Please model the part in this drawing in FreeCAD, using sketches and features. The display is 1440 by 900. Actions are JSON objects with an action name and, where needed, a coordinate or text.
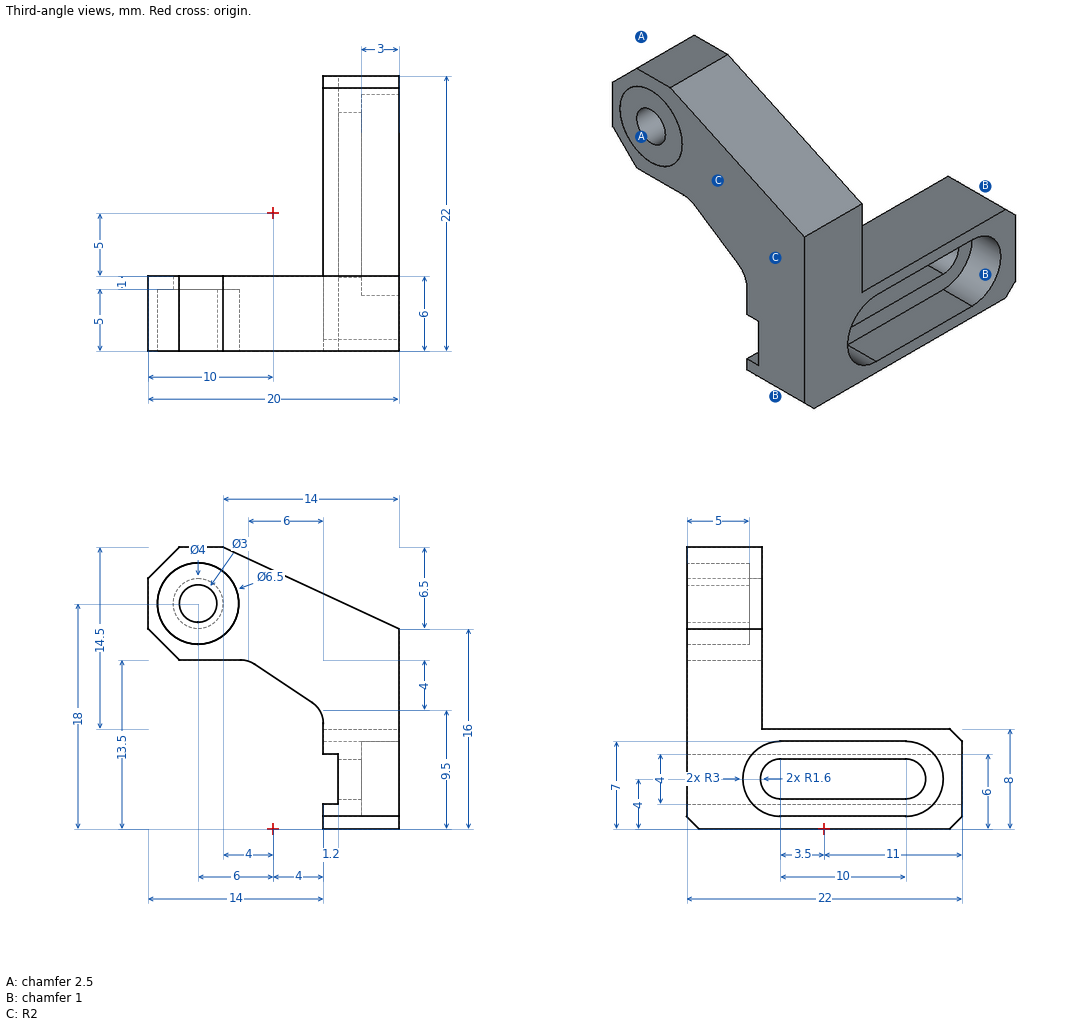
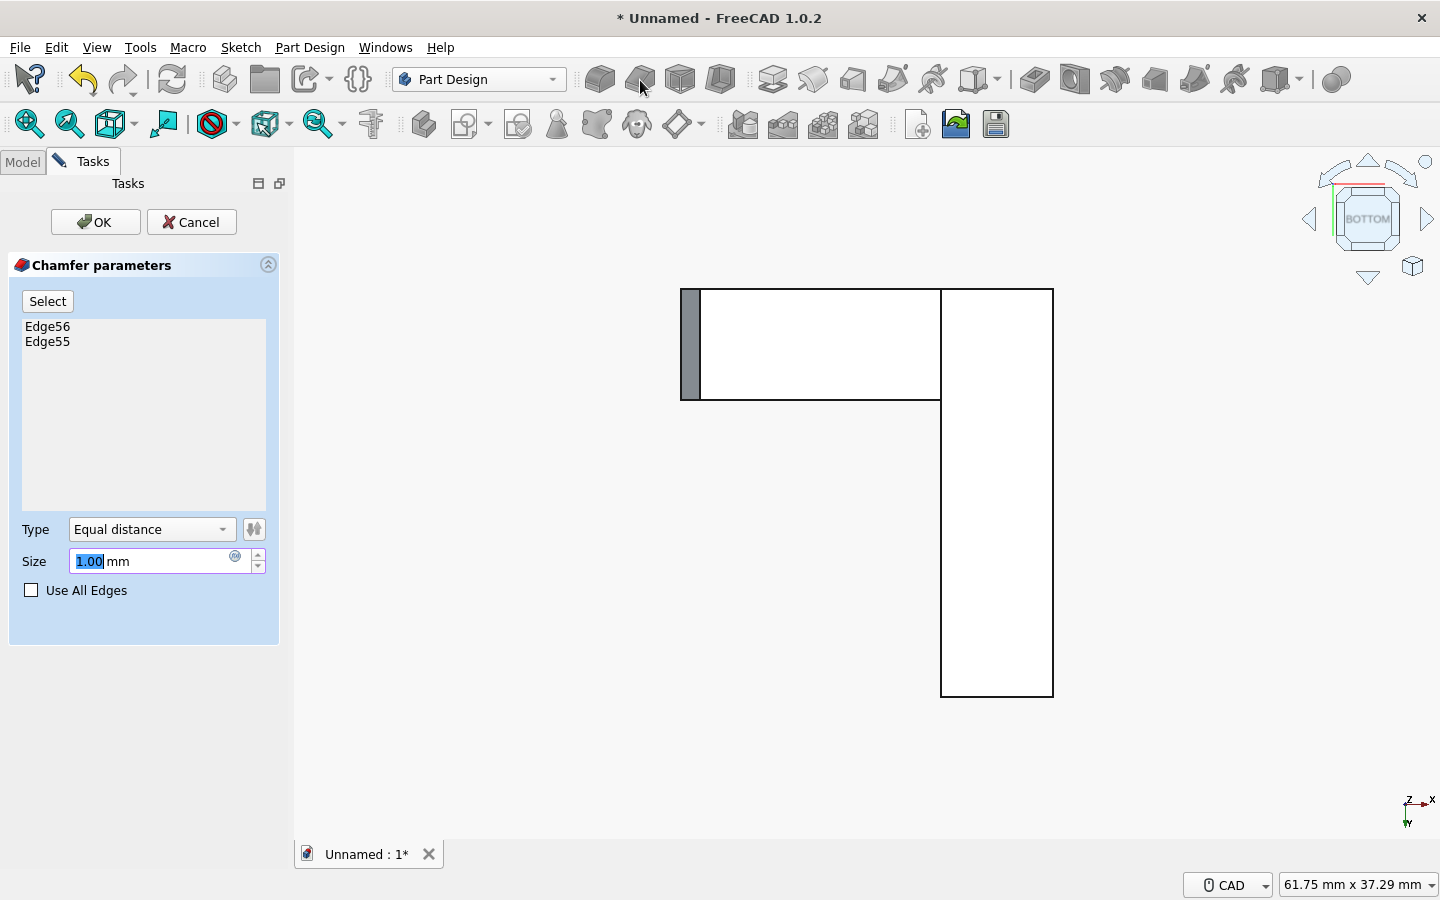
{"action": "type", "text": "2.5"}
{"action": "key", "text": "Tab"}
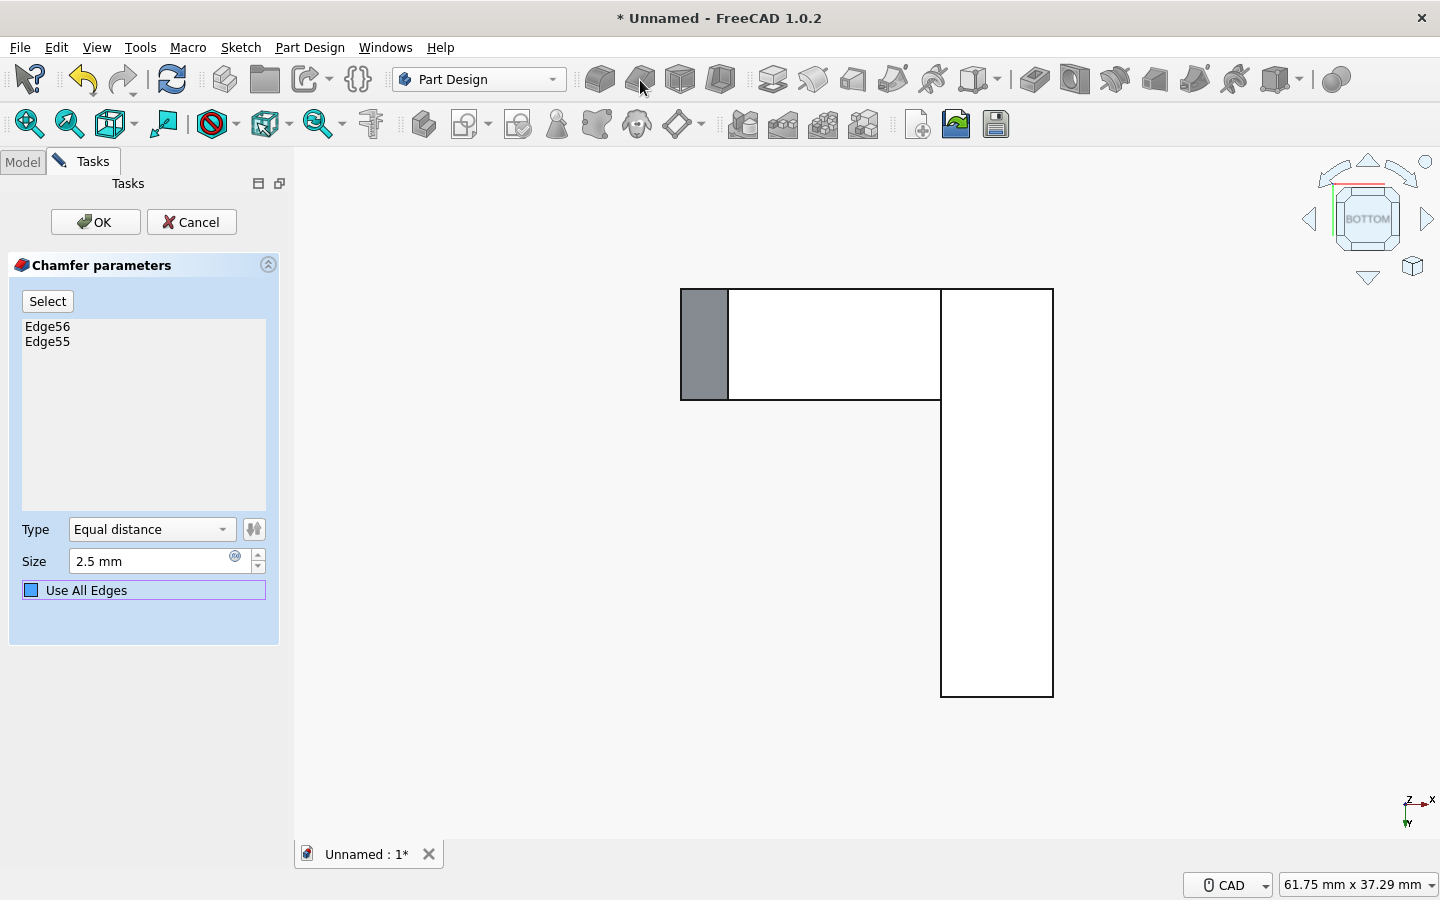
{"action": "left_click", "coordinate": [96, 222]}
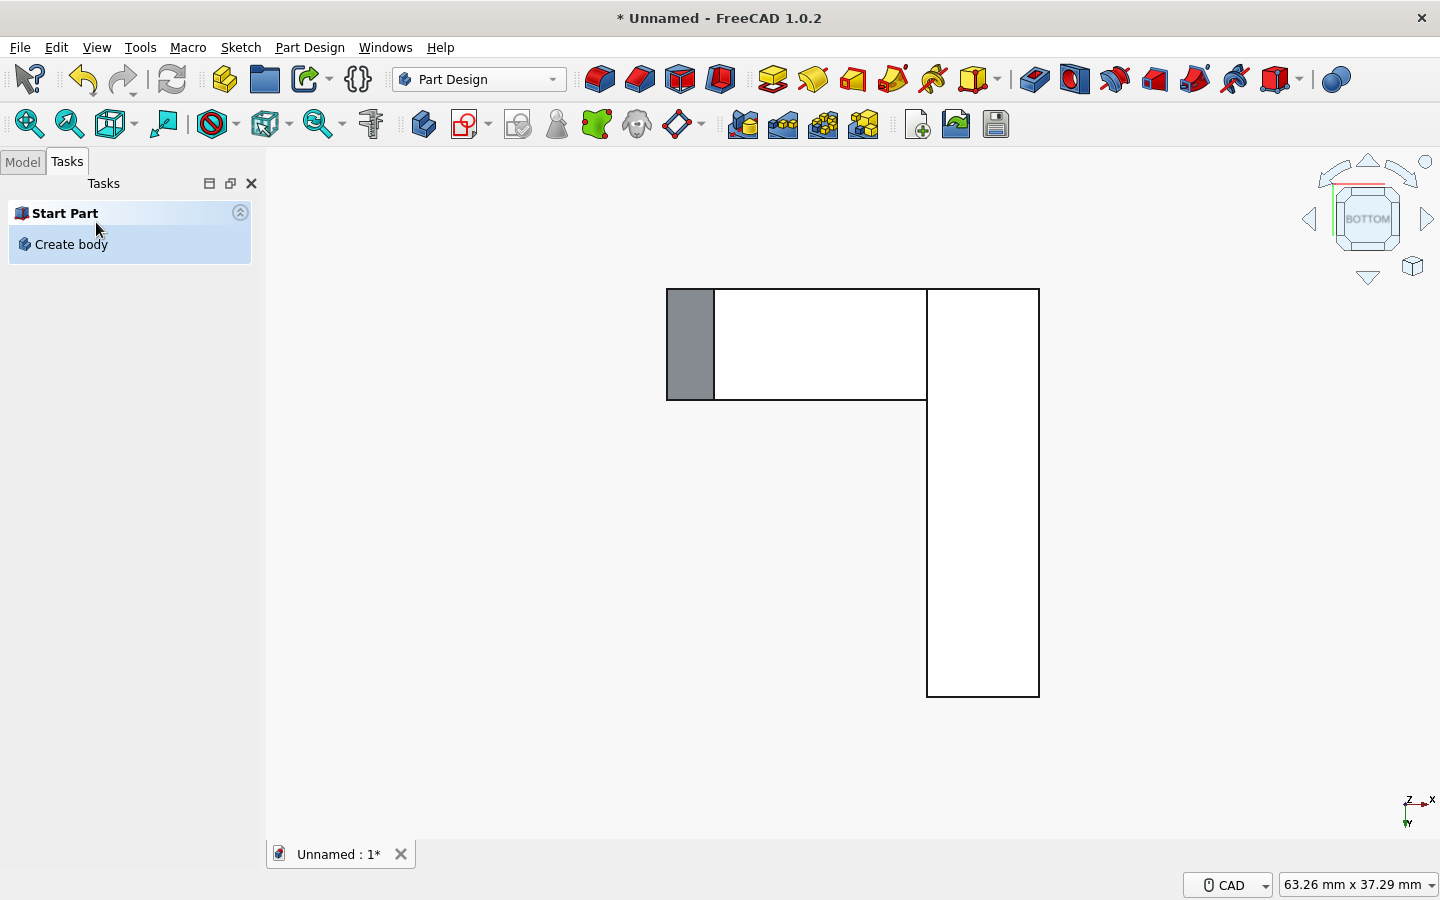
{"action": "left_click", "coordinate": [983, 288]}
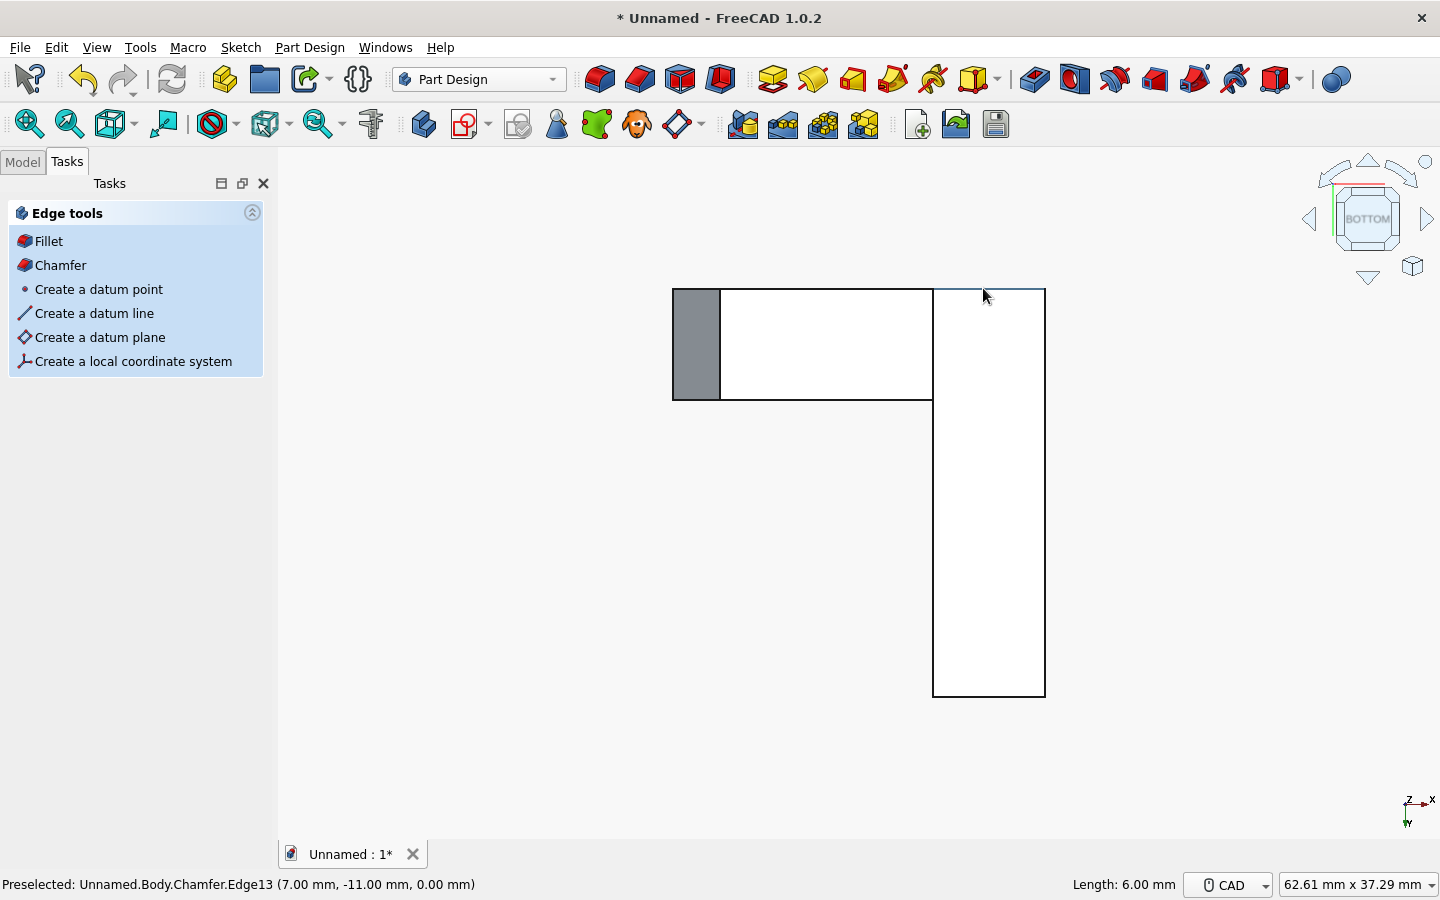
{"action": "left_click", "coordinate": [989, 696], "text": "ctrl"}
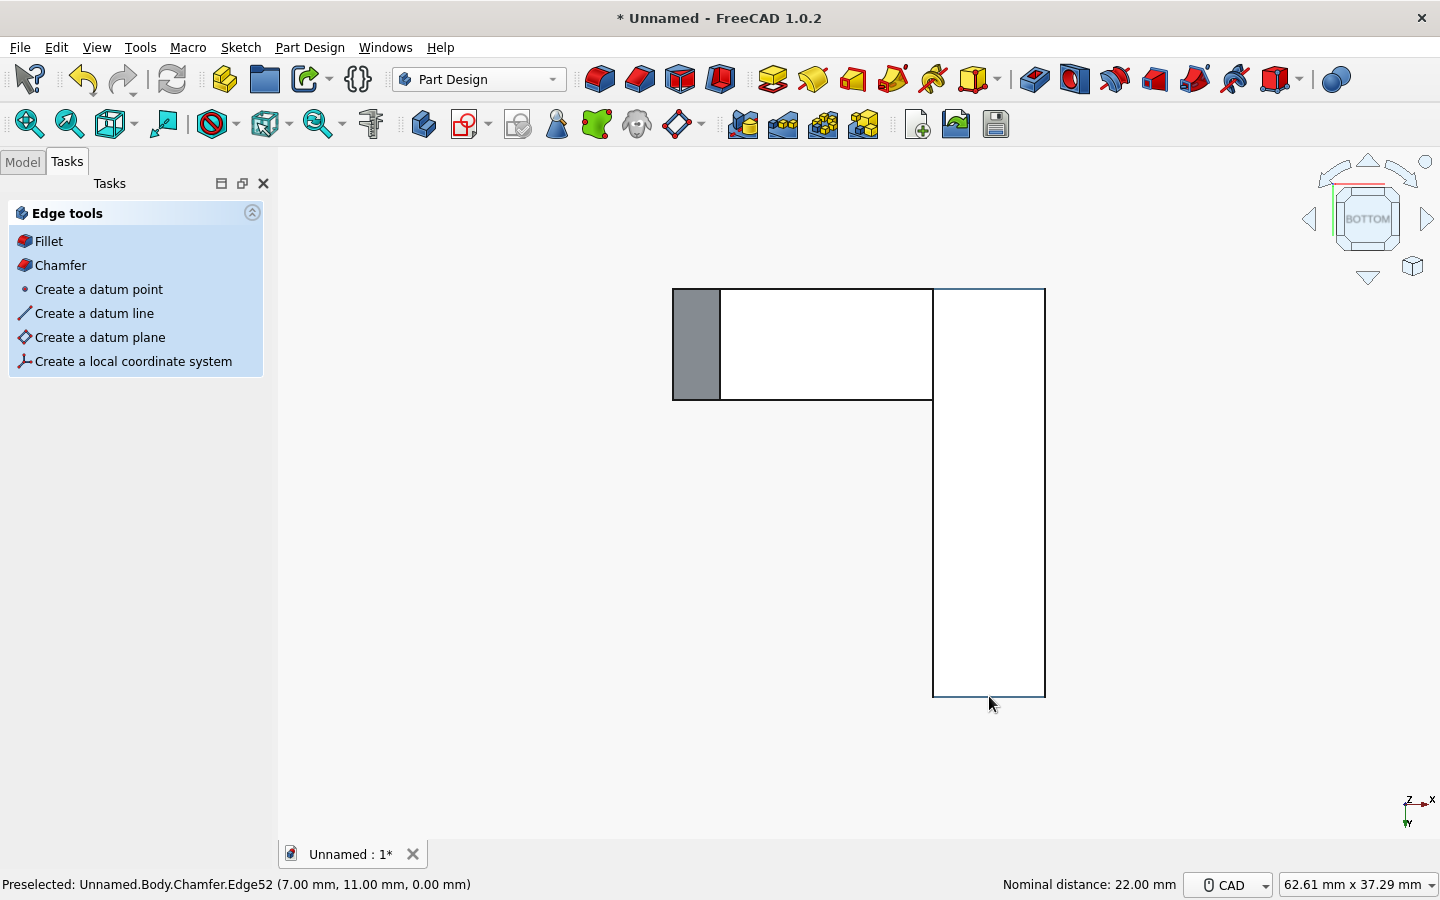
{"action": "key", "text": "0"}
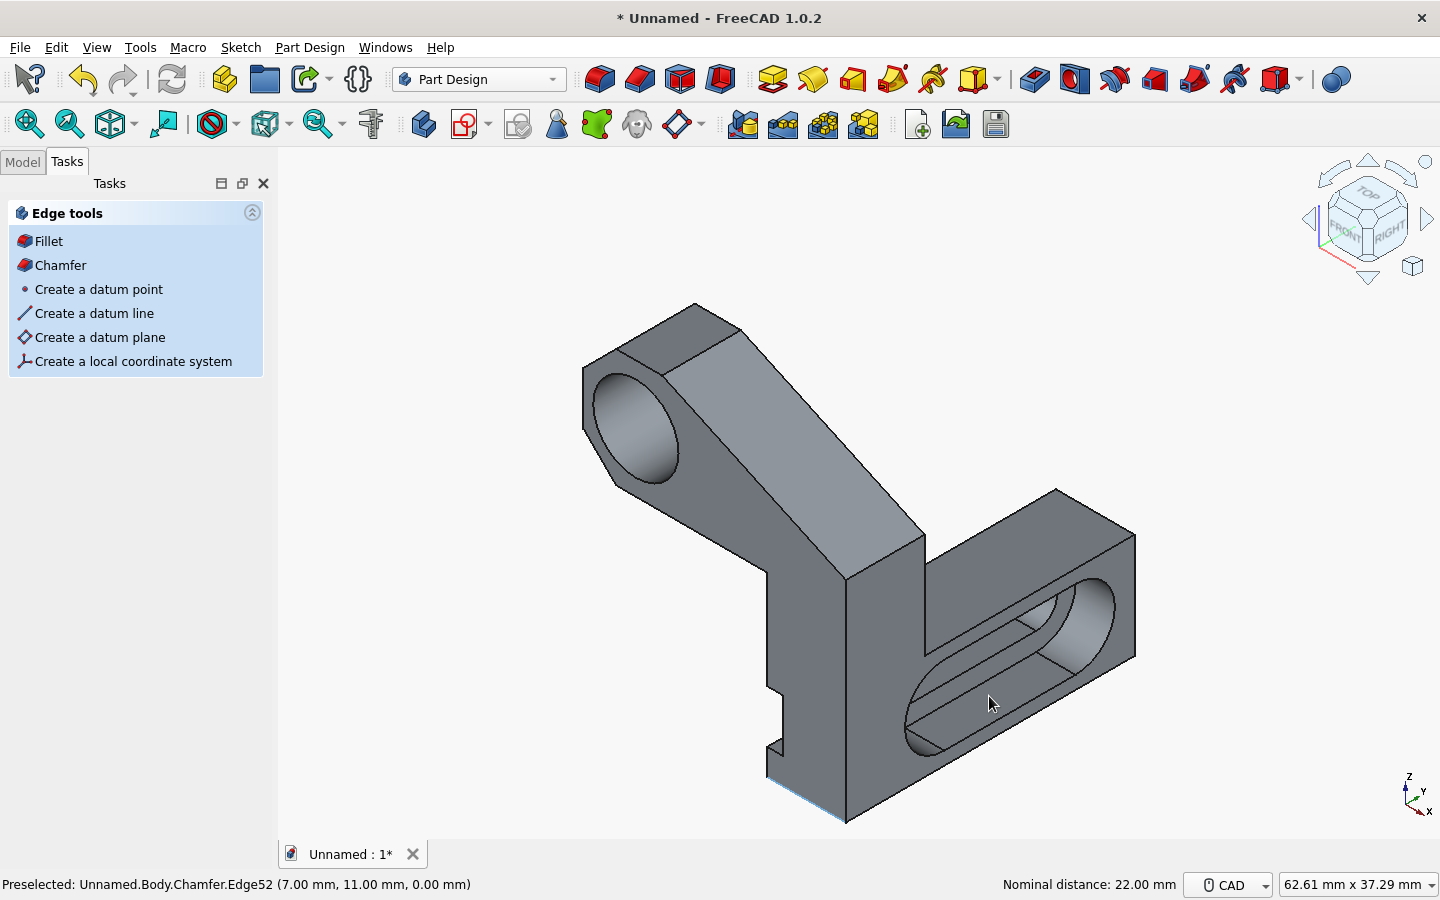
{"action": "key", "text": "2"}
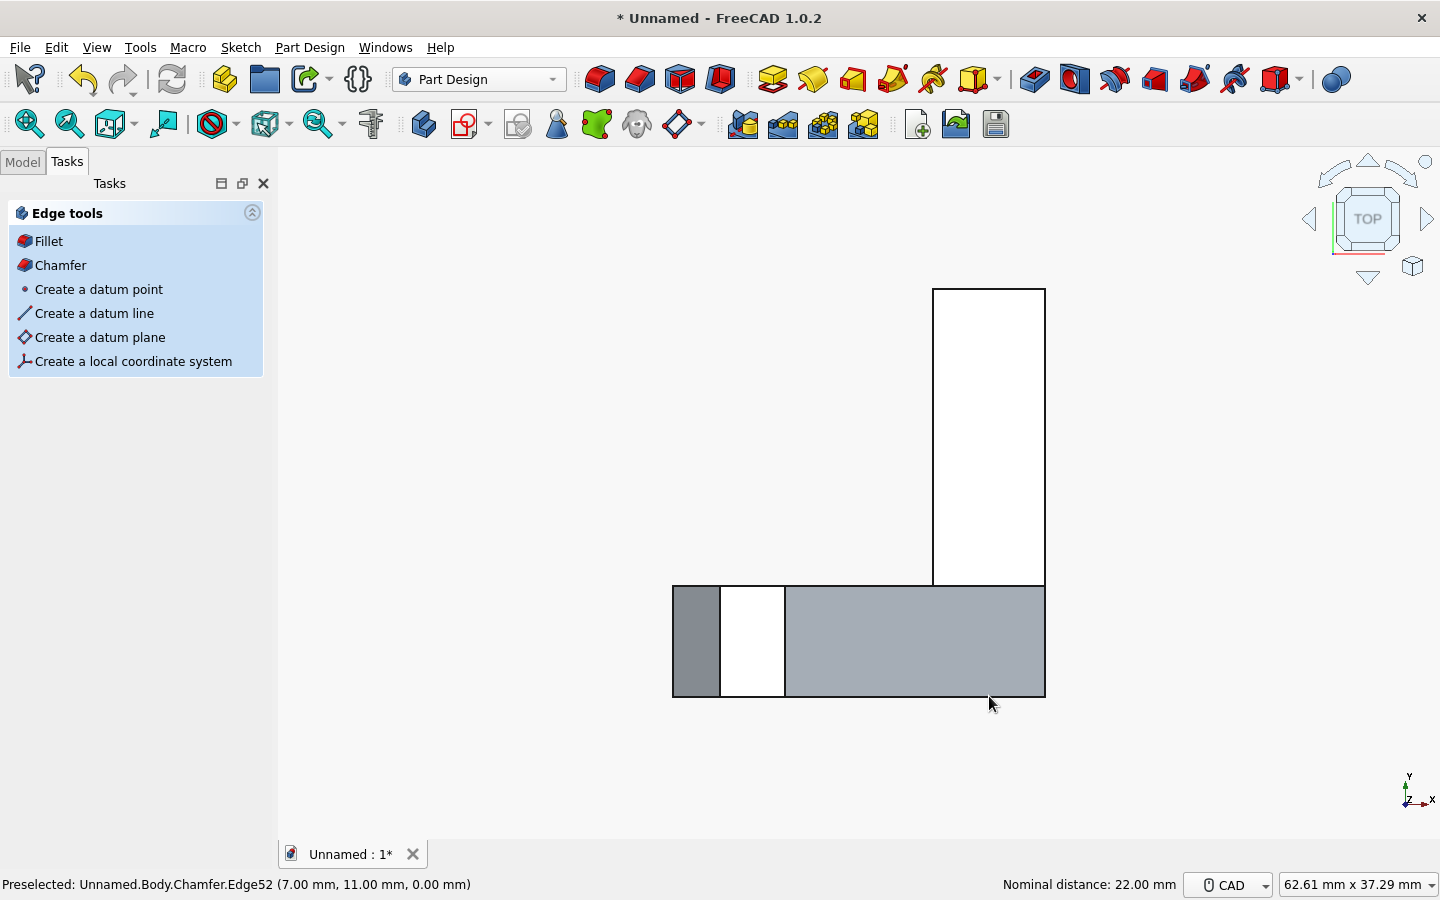
{"action": "left_click", "coordinate": [989, 288], "text": "ctrl"}